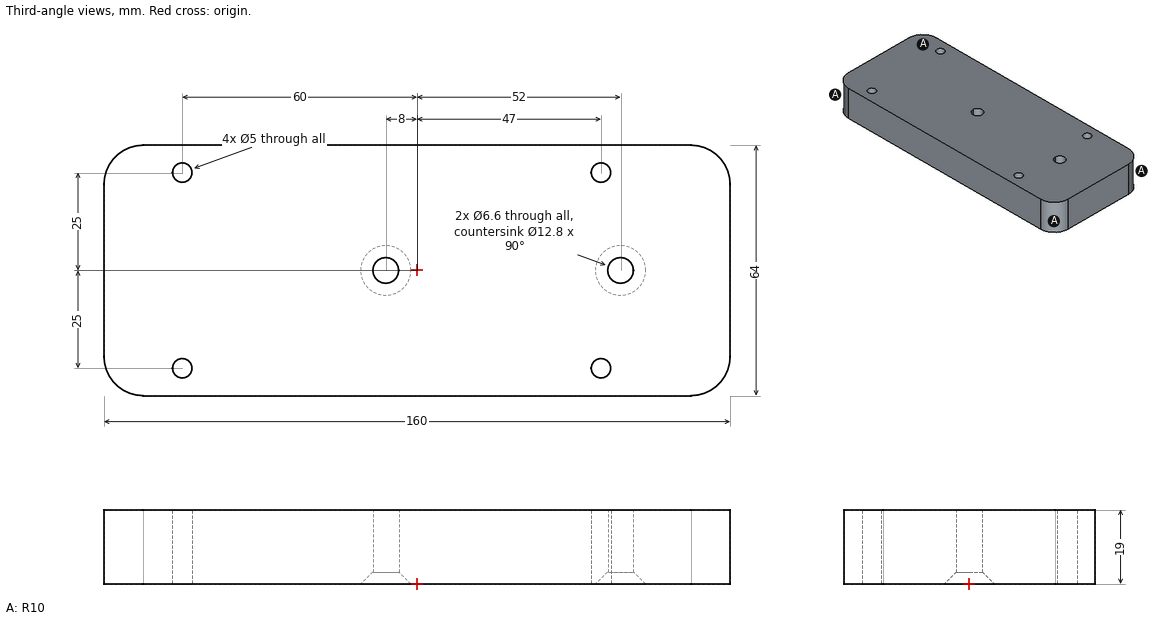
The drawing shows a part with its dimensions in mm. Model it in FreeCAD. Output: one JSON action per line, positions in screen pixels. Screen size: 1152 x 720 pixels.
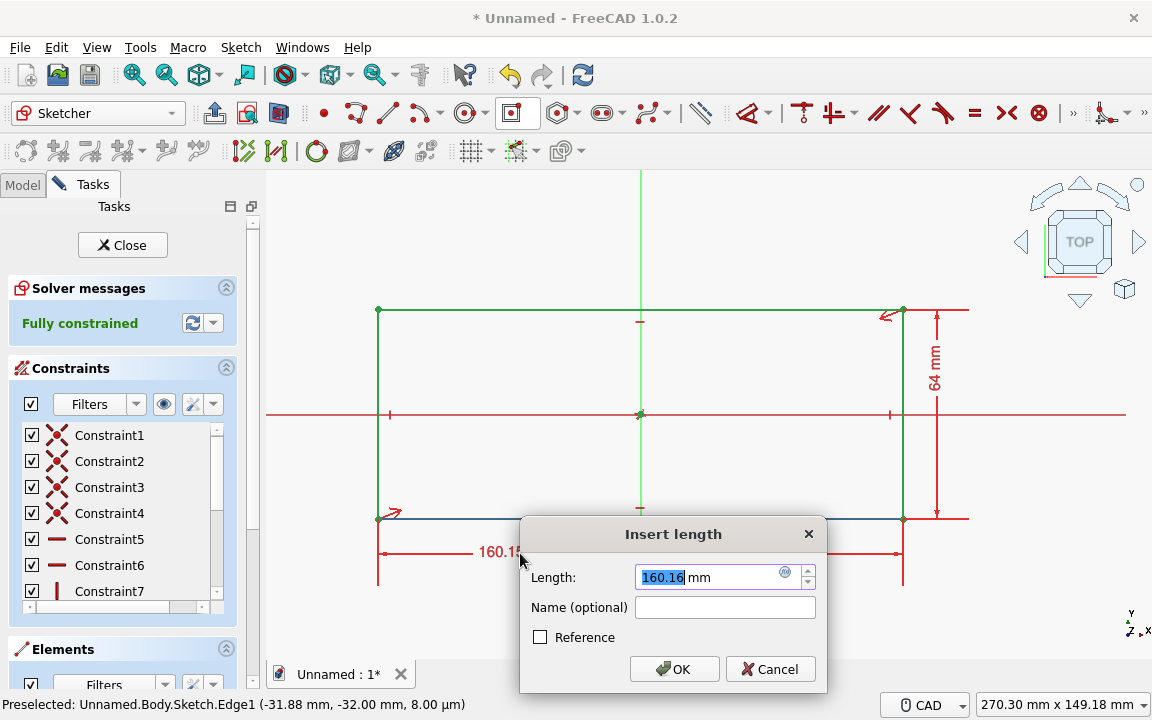
{"action": "type", "text": "160"}
{"action": "key", "text": "Return"}
{"action": "key", "text": "Escape"}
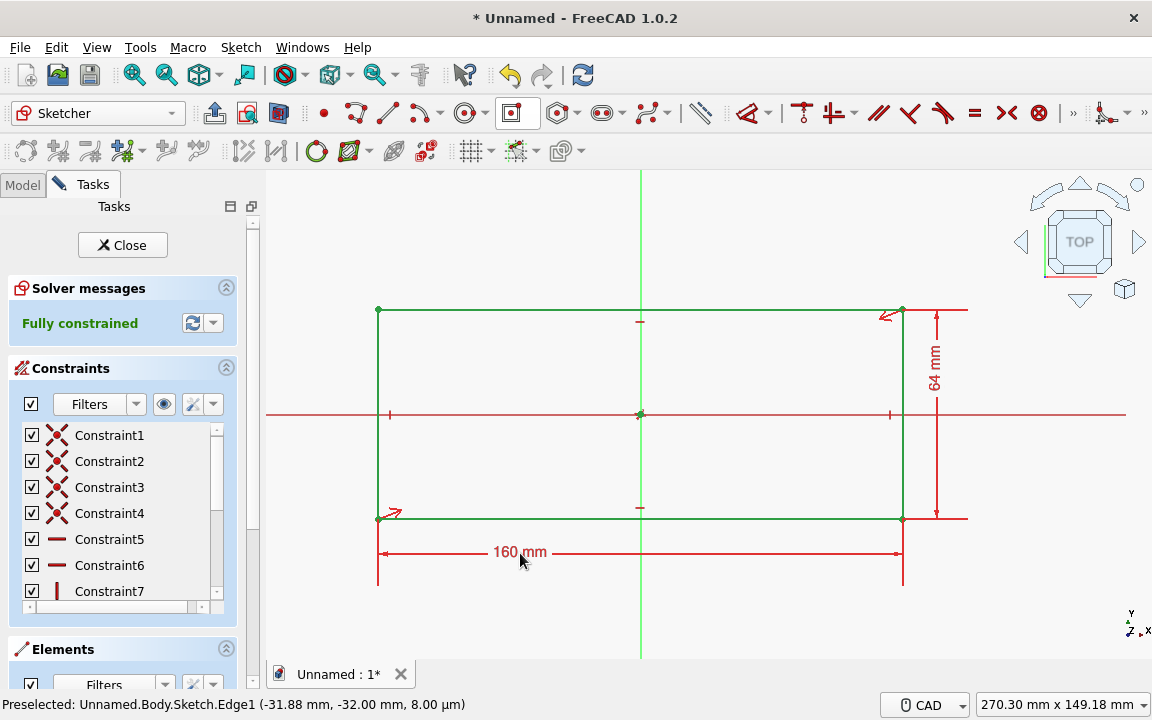
{"action": "left_click", "coordinate": [123, 245]}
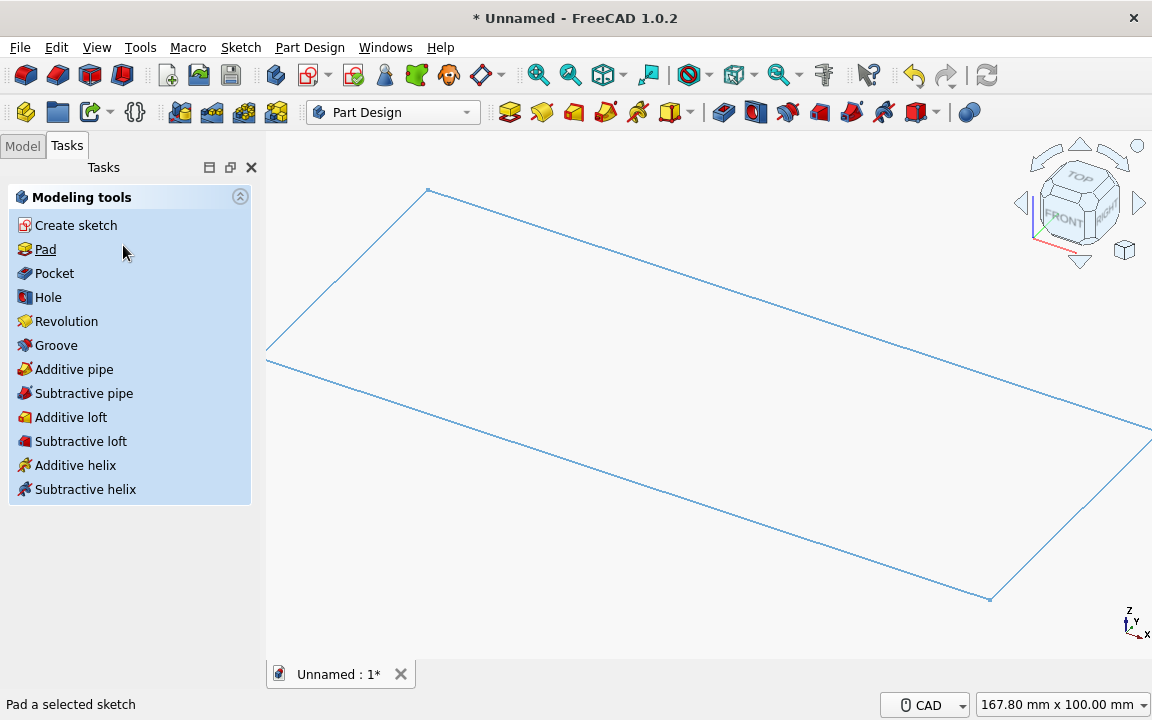
{"action": "left_click", "coordinate": [510, 112]}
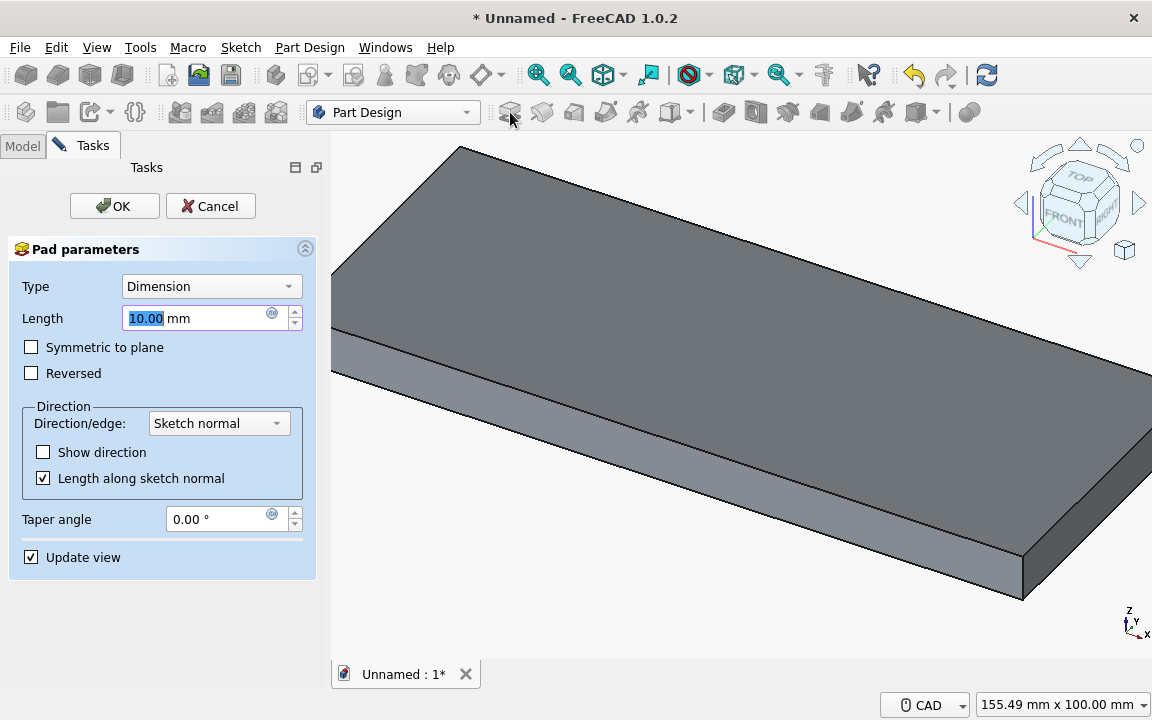
{"action": "type", "text": "19"}
{"action": "key", "text": "Tab"}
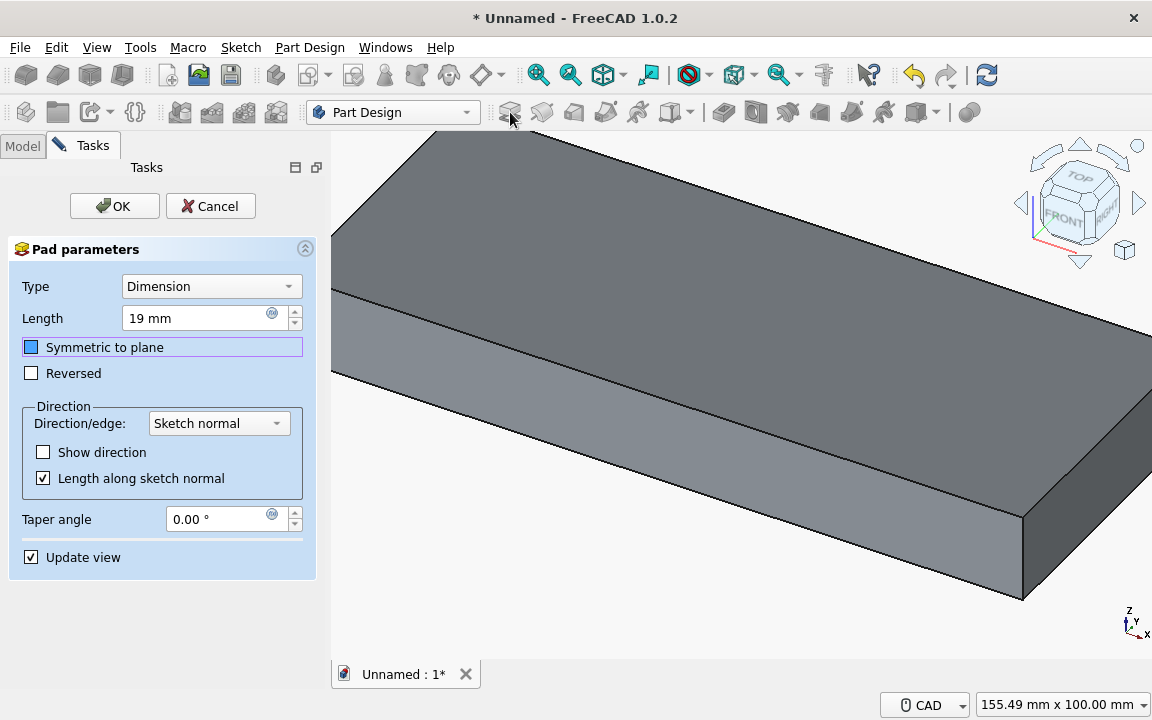
{"action": "left_click", "coordinate": [115, 206]}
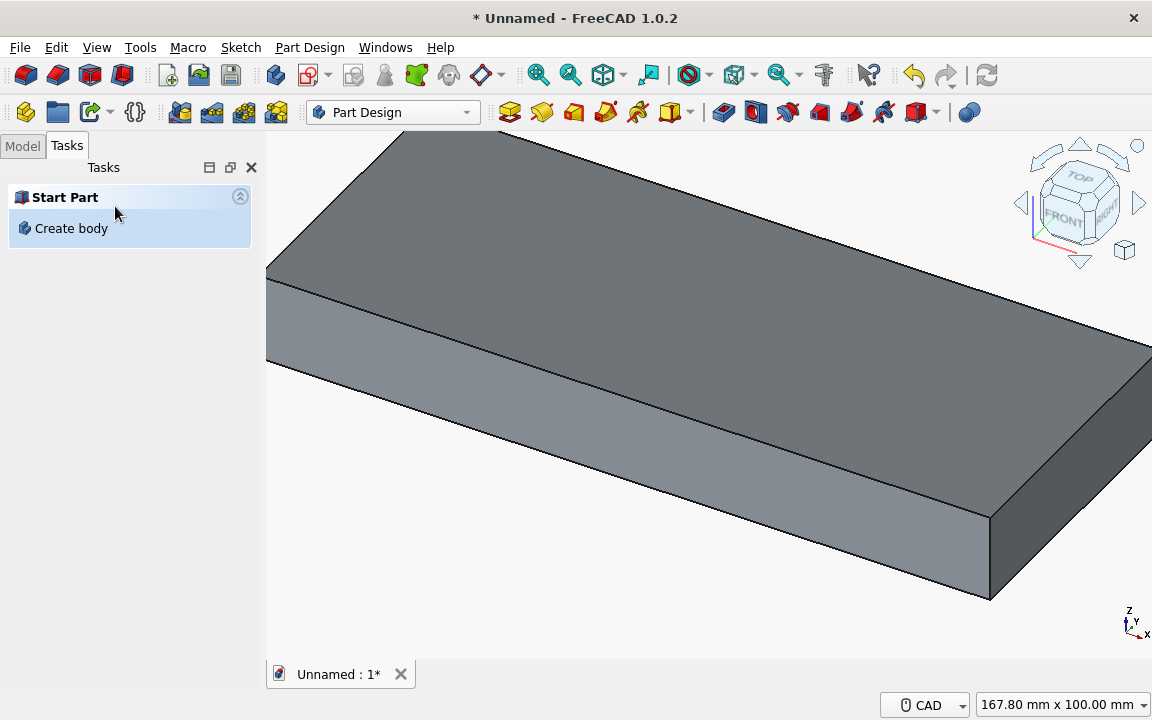
{"action": "left_click", "coordinate": [540, 76]}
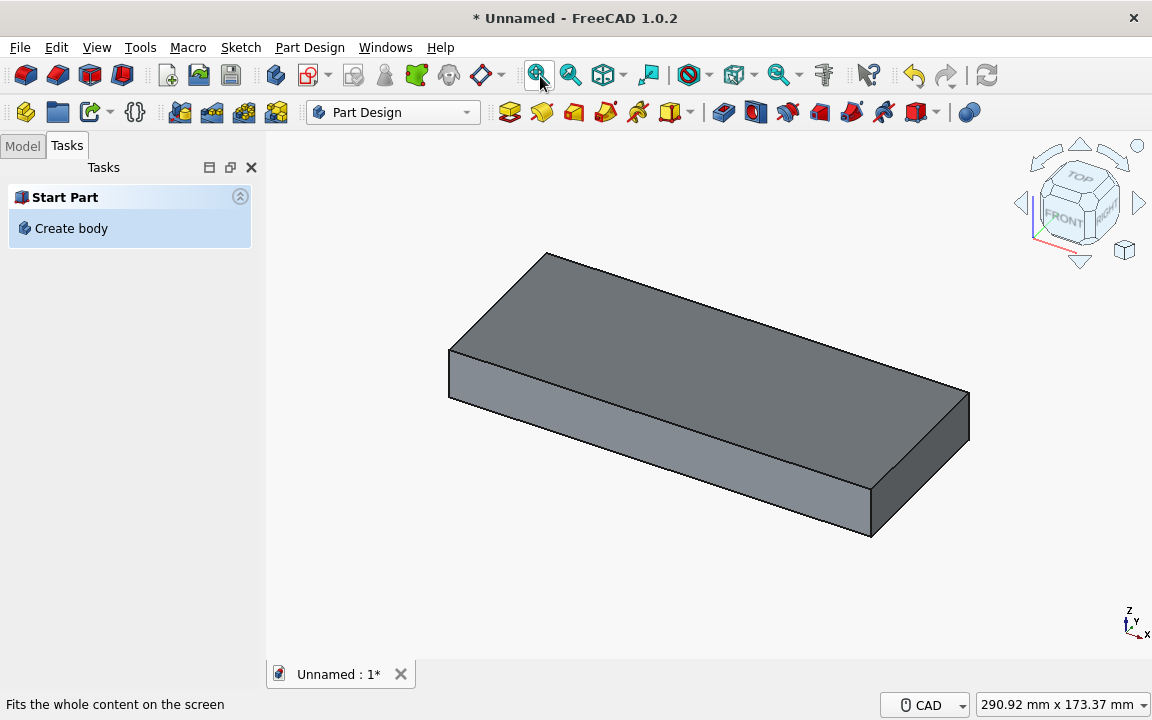
{"action": "left_click", "coordinate": [871, 512]}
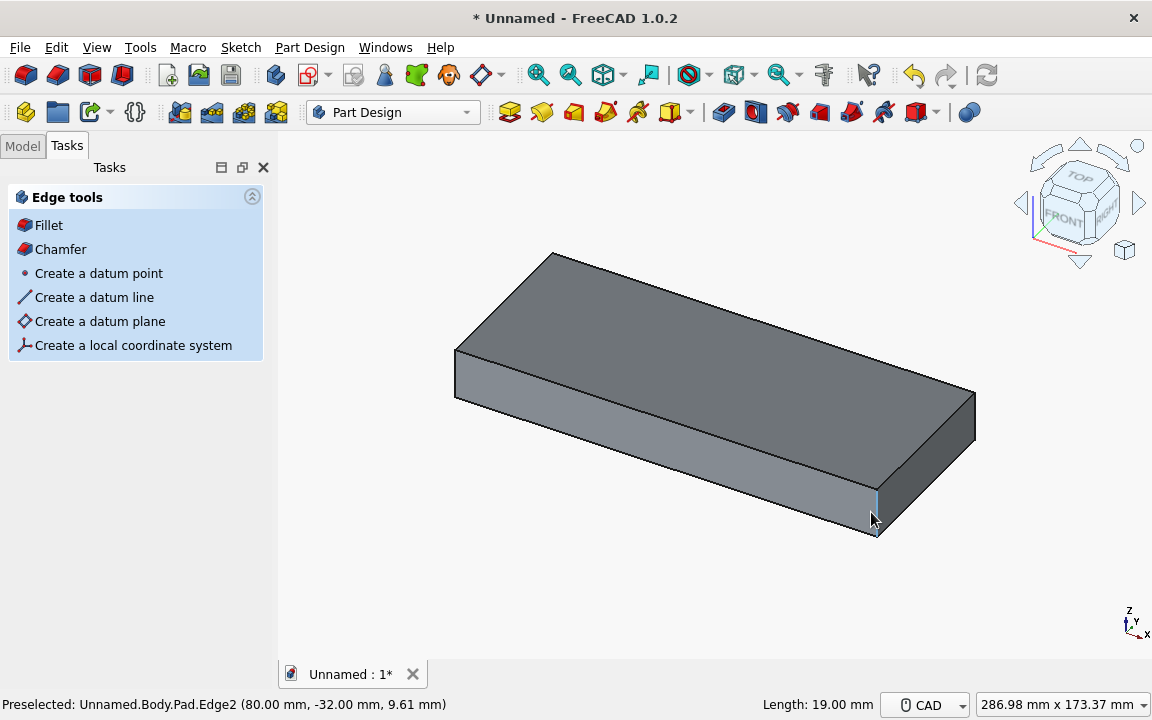
{"action": "key", "text": "0"}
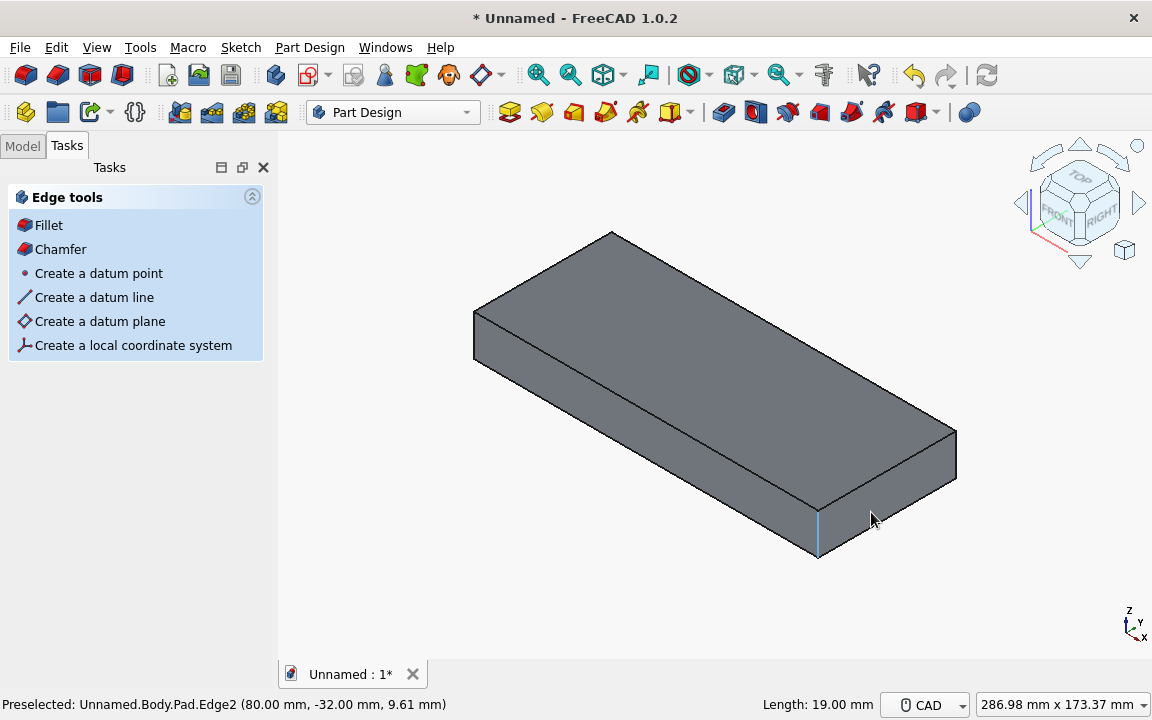
{"action": "key", "text": "2"}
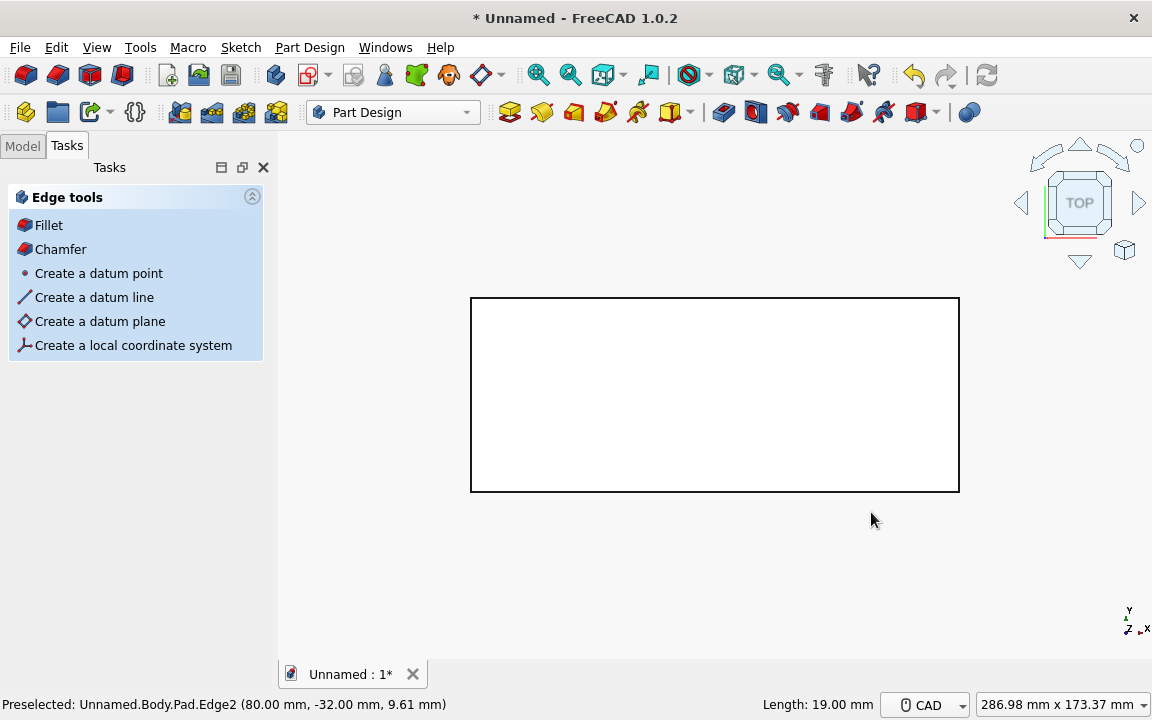
{"action": "key", "text": "1"}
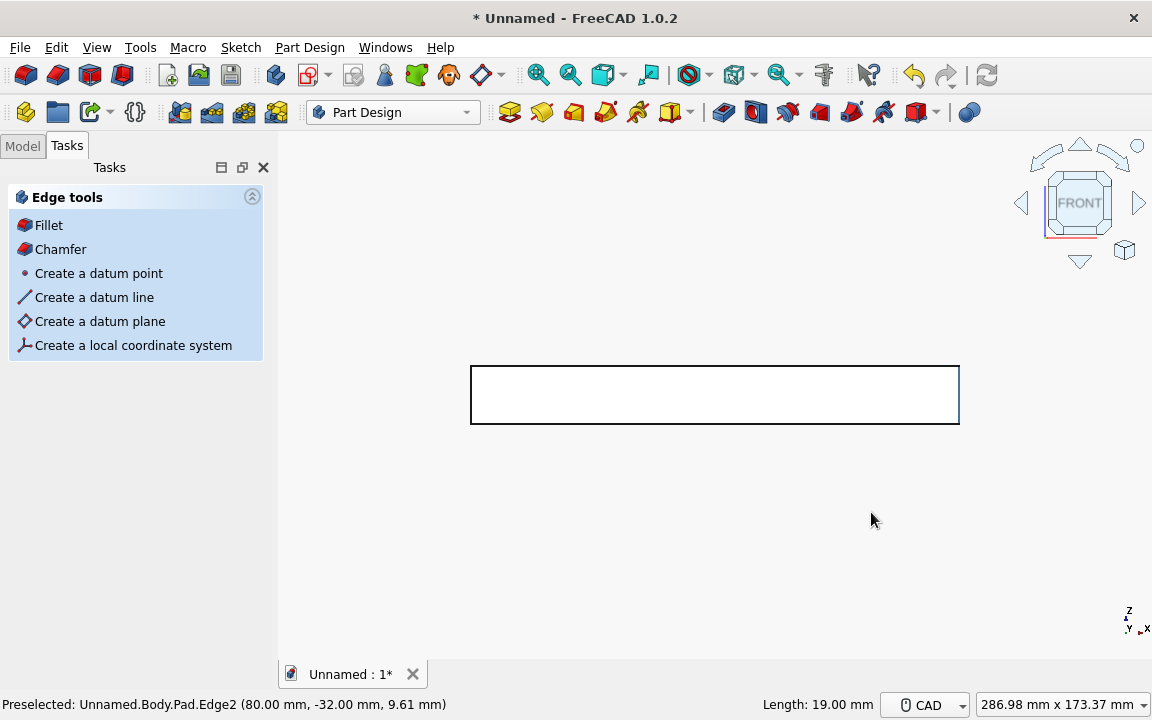
{"action": "left_click", "coordinate": [471, 394], "text": "ctrl"}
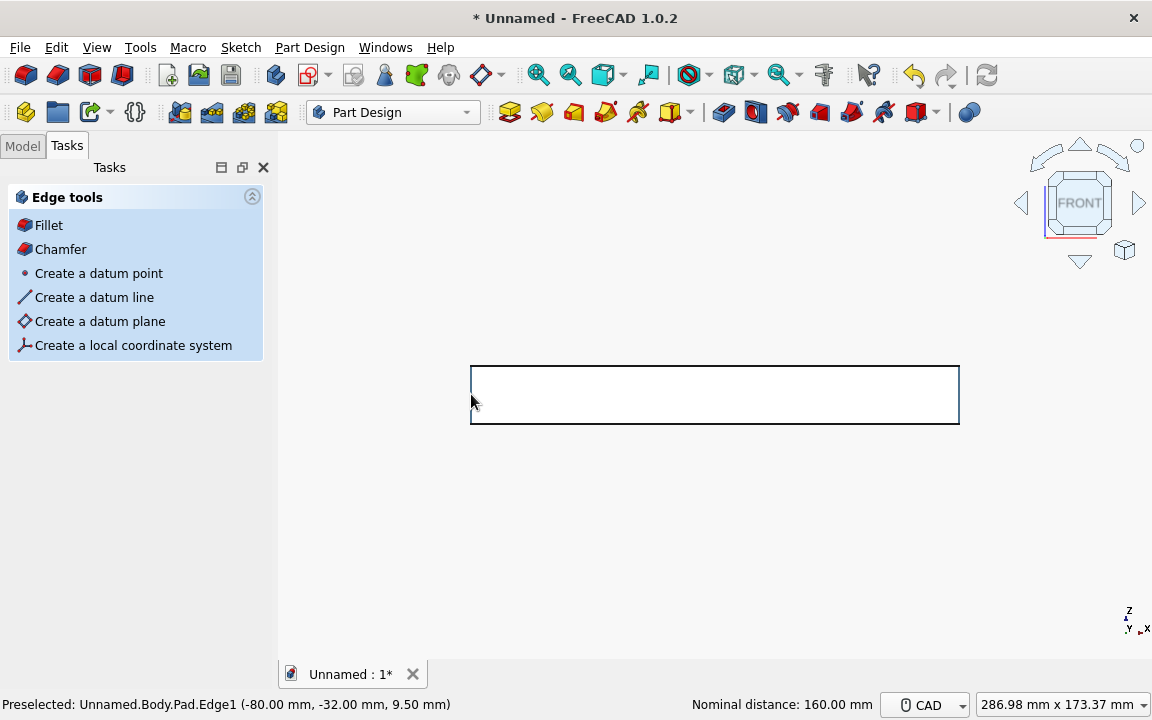
{"action": "key", "text": "3"}